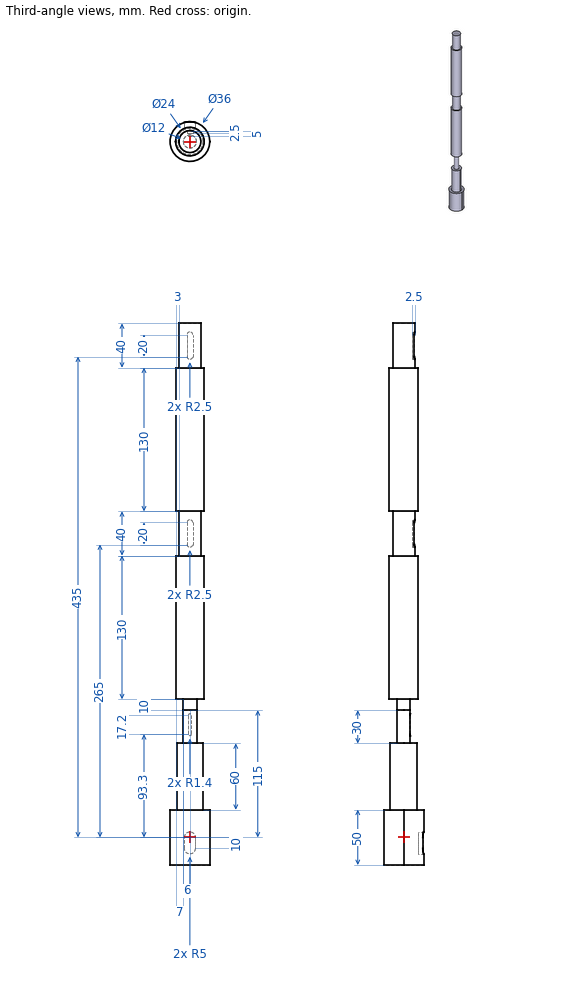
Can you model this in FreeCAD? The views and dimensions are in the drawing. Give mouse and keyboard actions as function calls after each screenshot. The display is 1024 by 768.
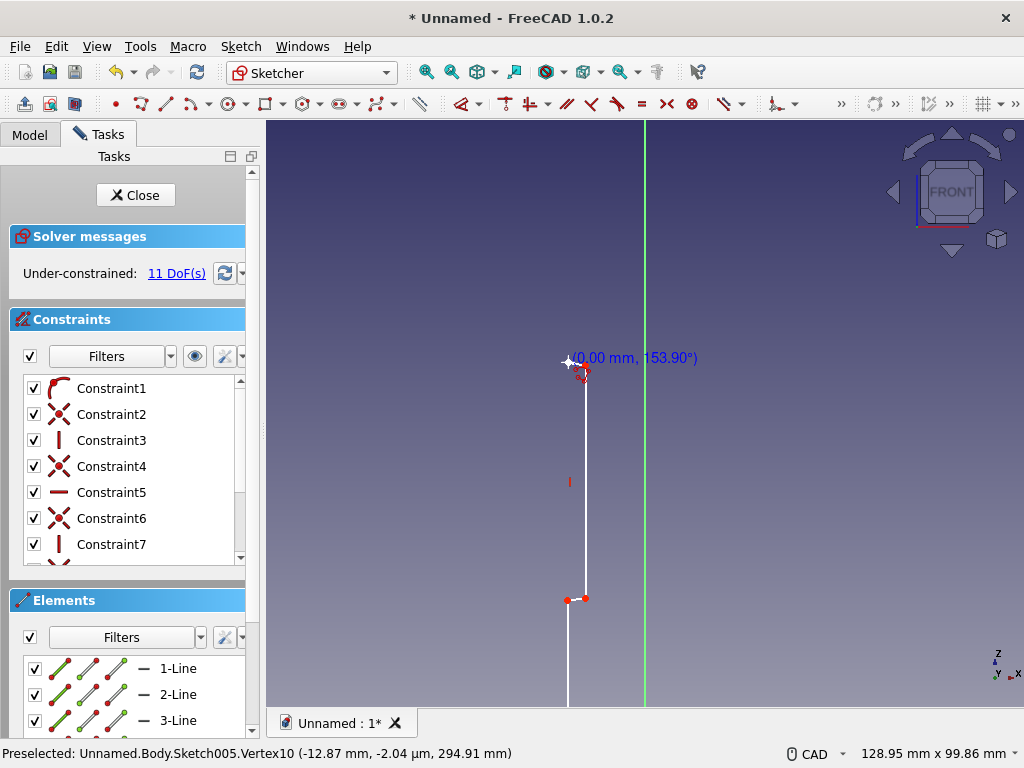
scroll(572, 364, down, 10)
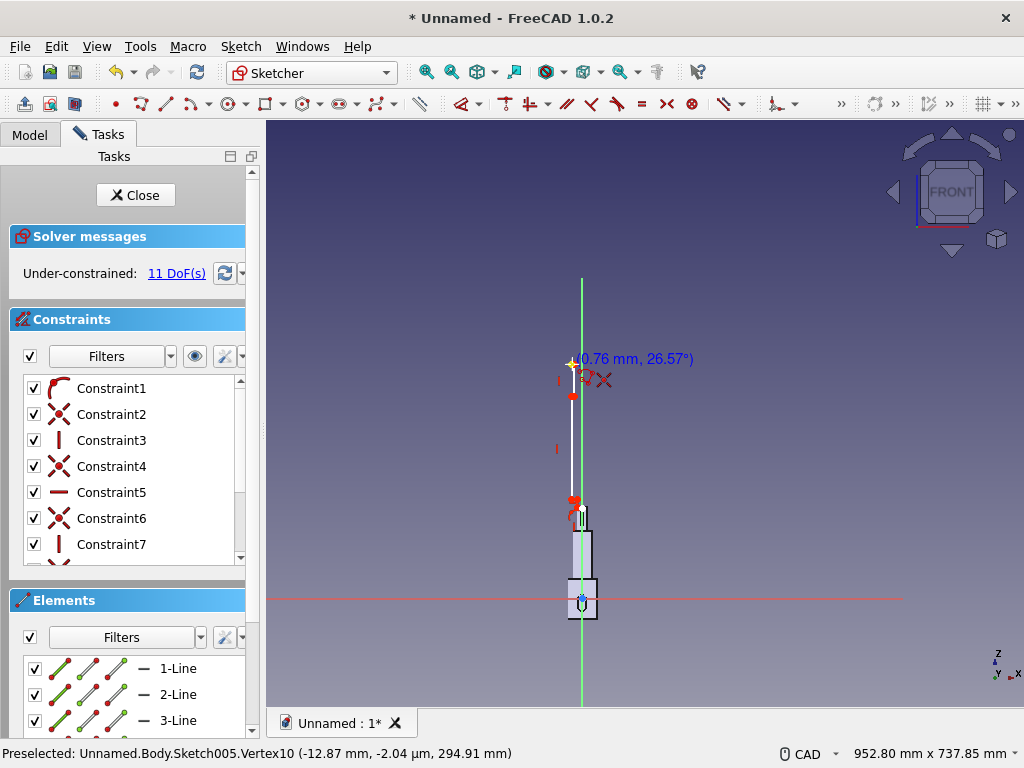
scroll(572, 261, up, 3)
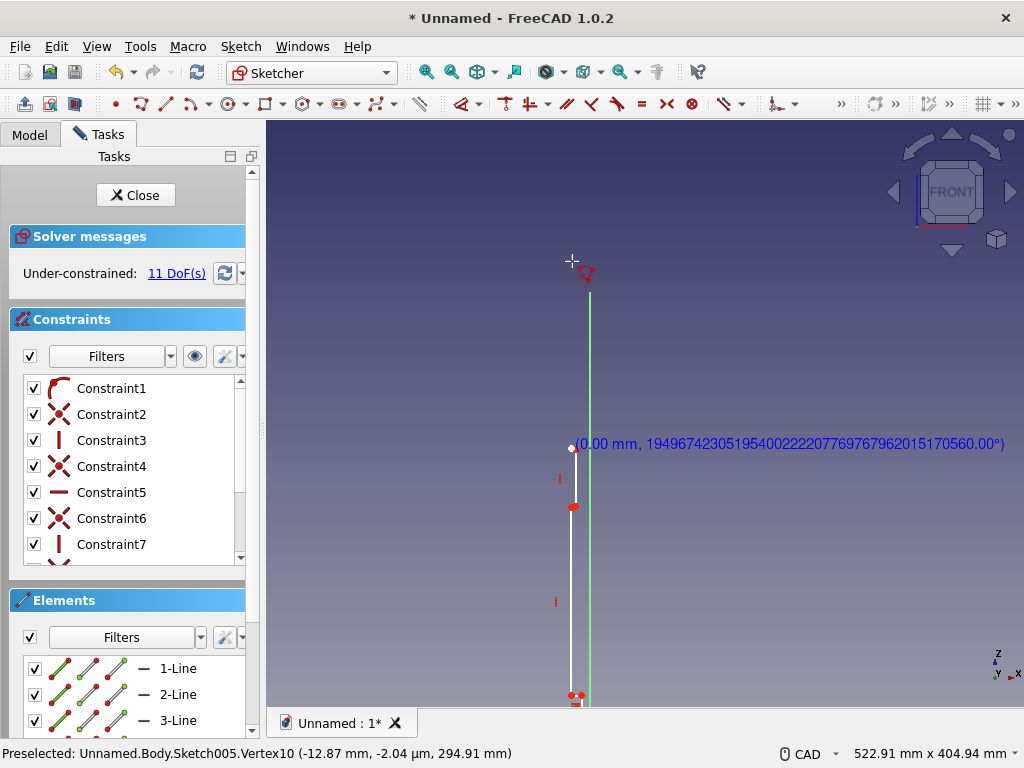
click(571, 261)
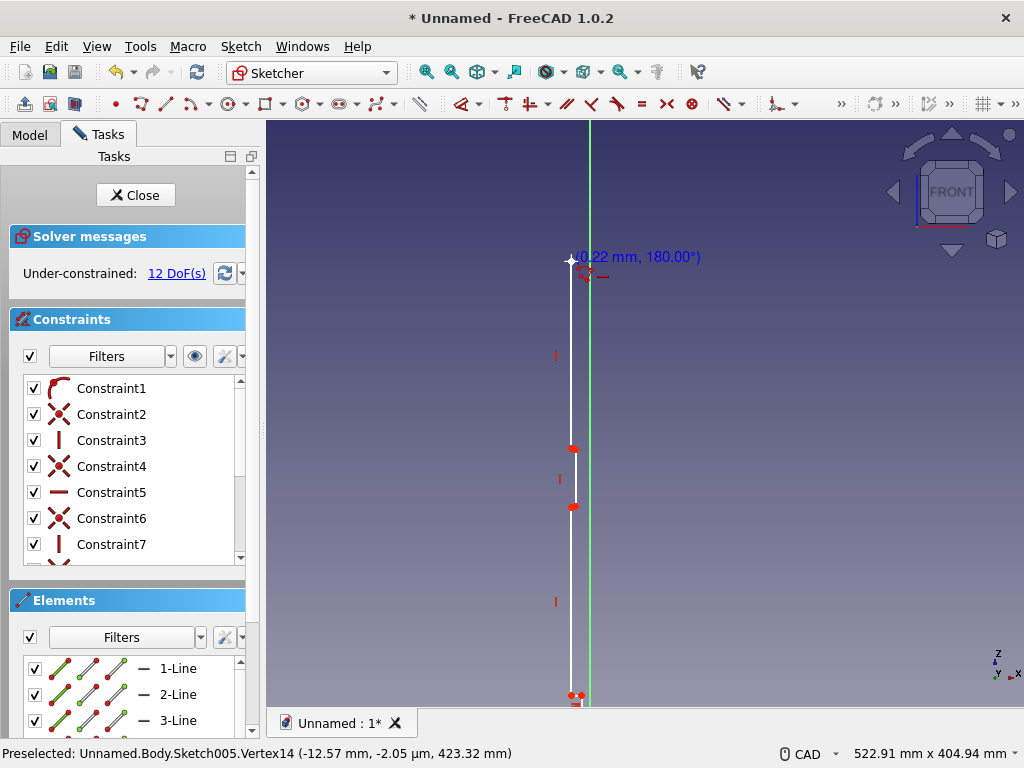
scroll(576, 261, up, 7)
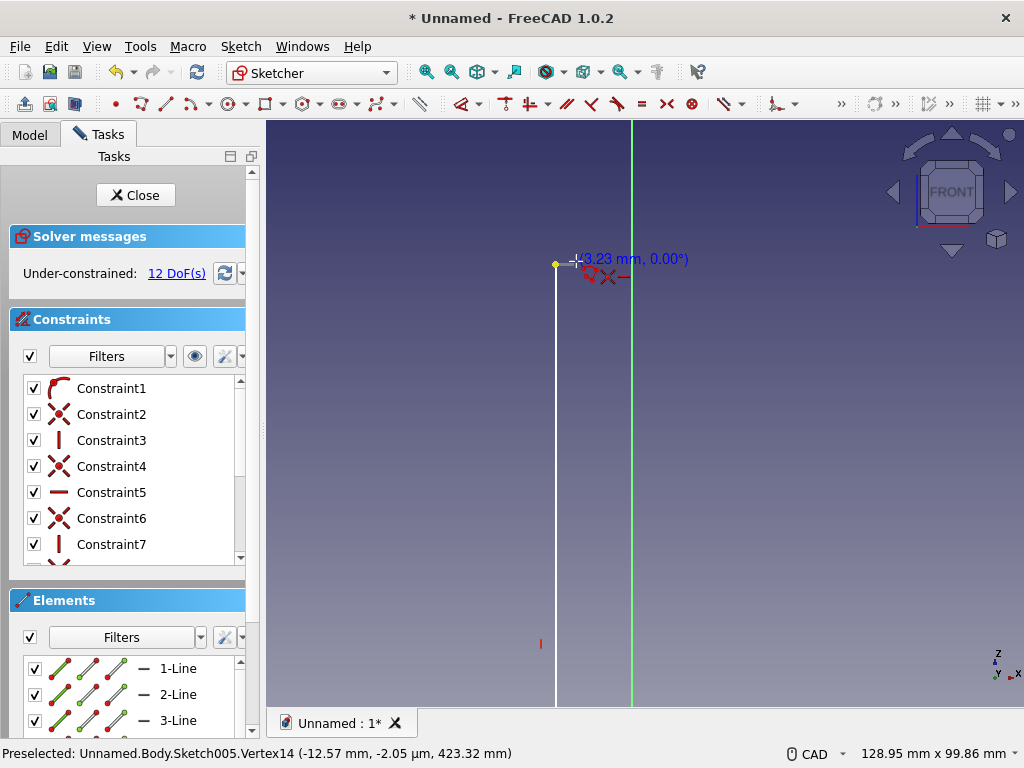
click(574, 260)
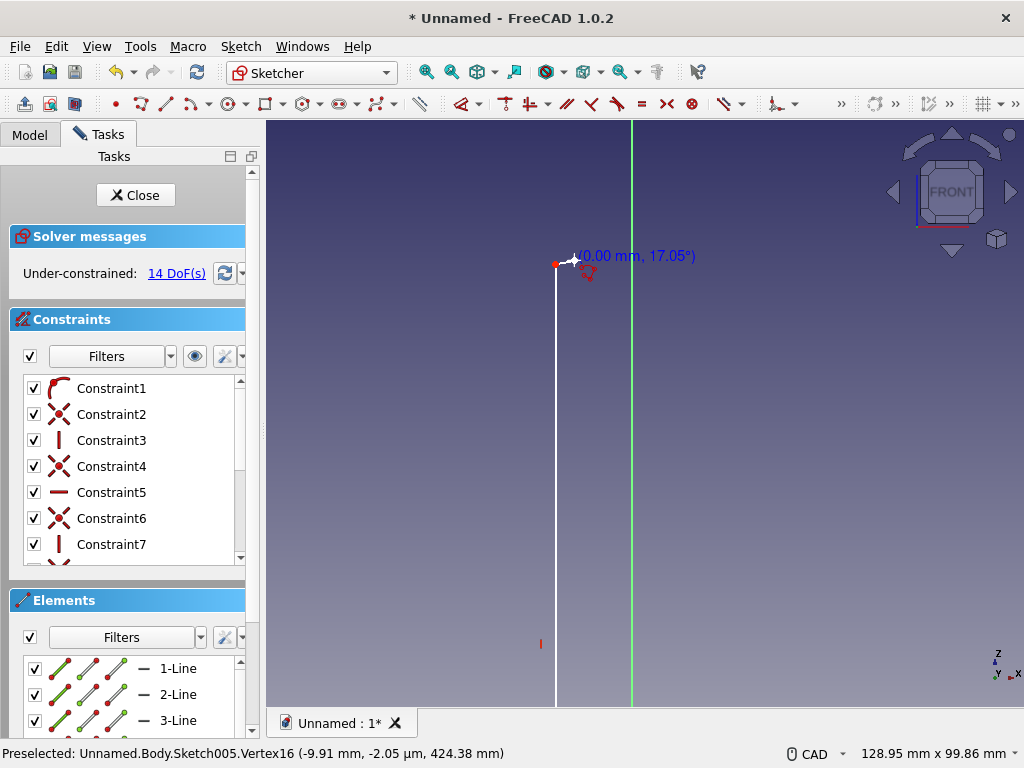
scroll(574, 261, down, 10)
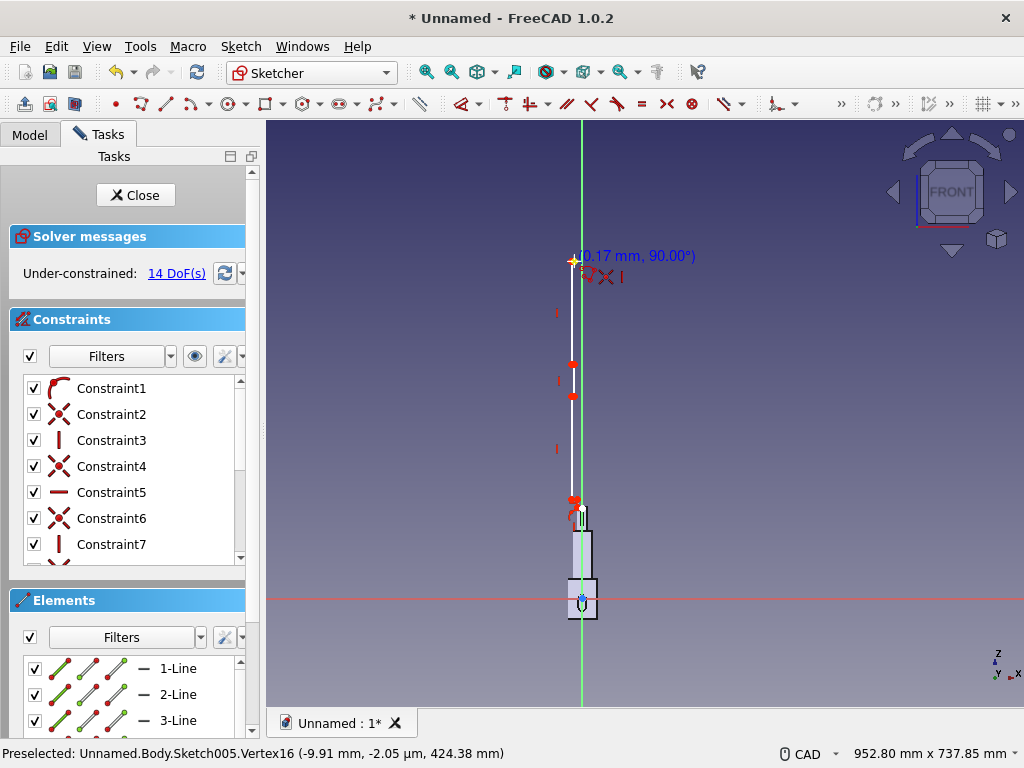
scroll(574, 229, up, 4)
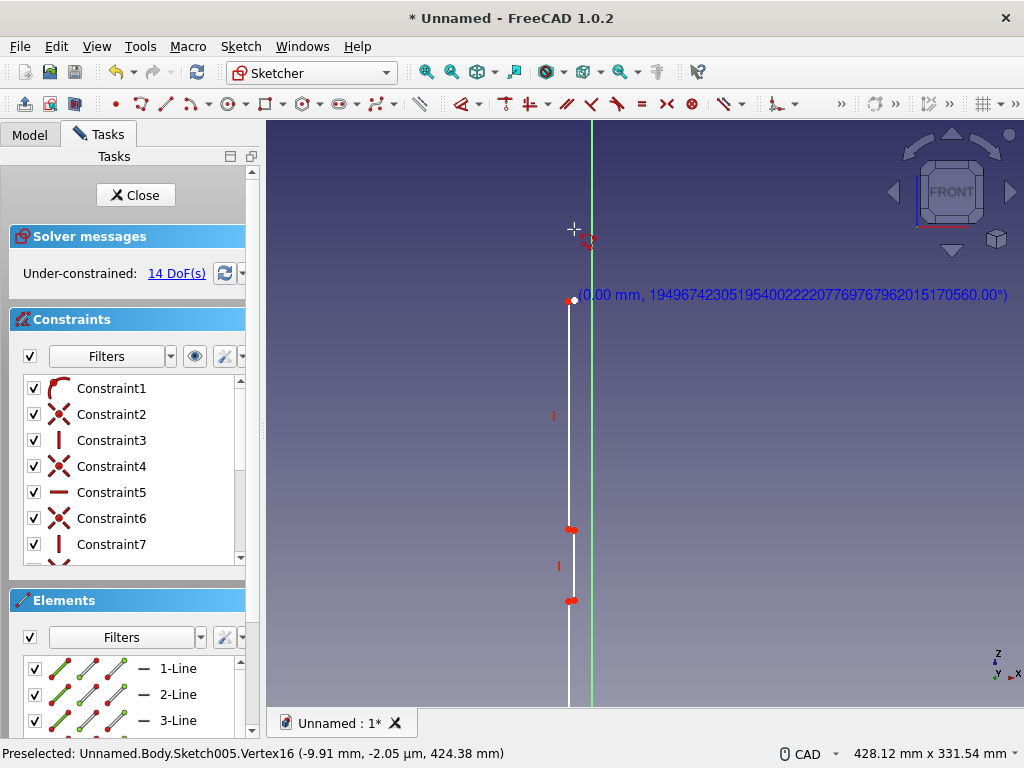
click(574, 229)
click(583, 229)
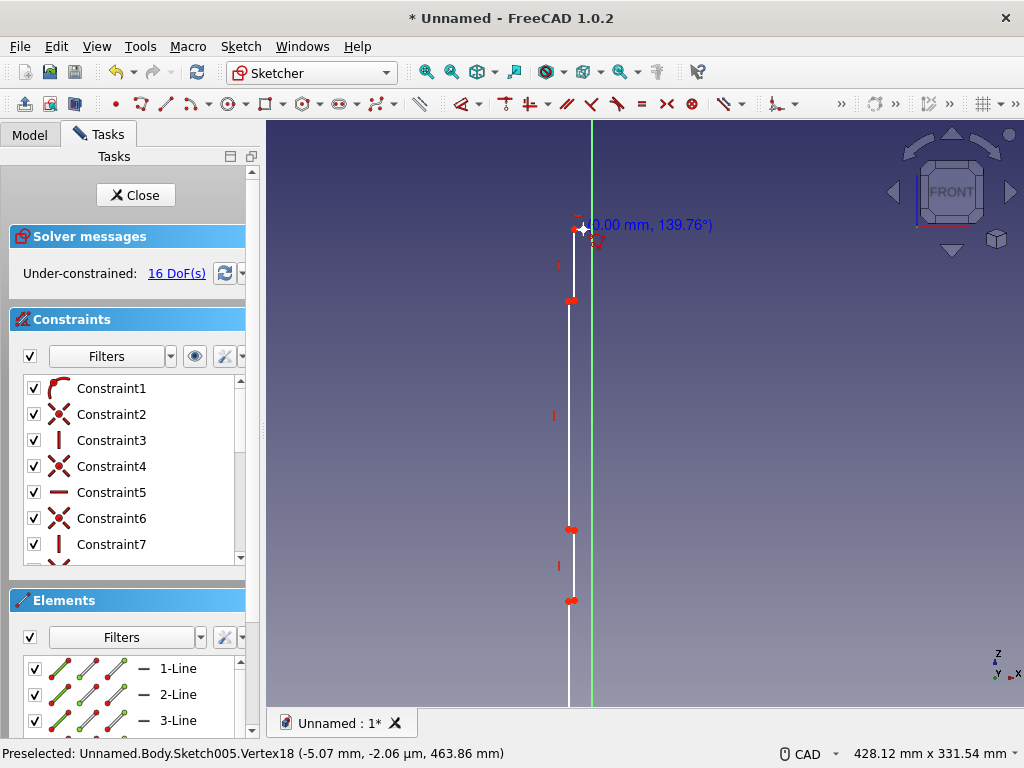
scroll(573, 228, down, 4)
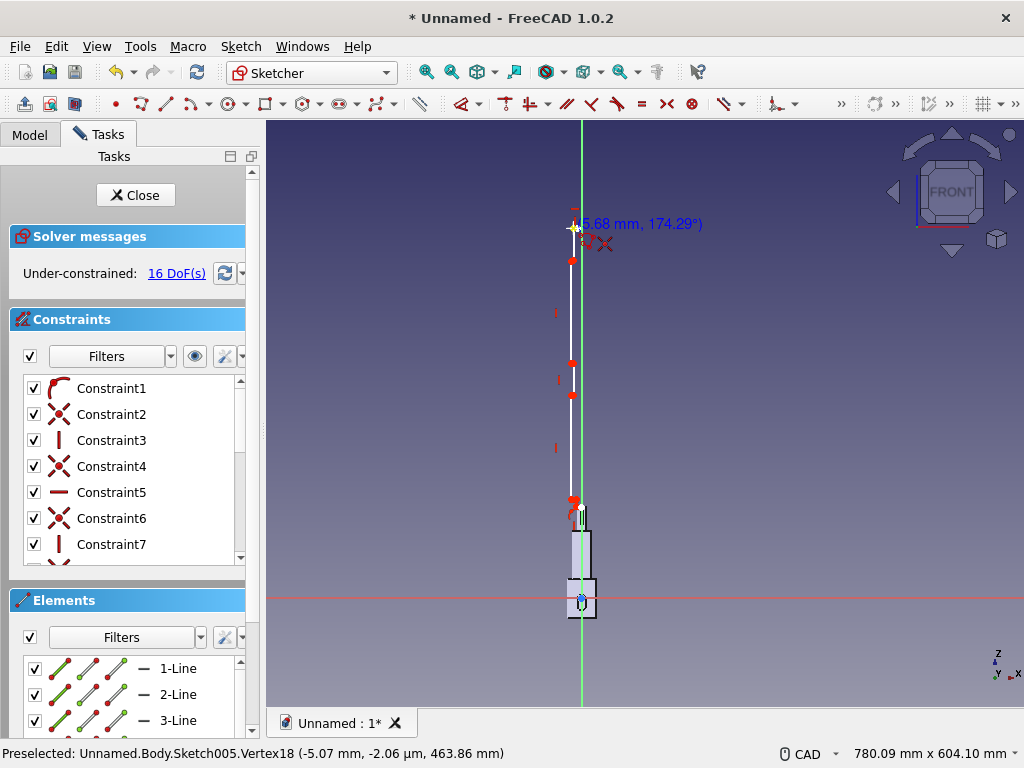
scroll(582, 507, up, 10)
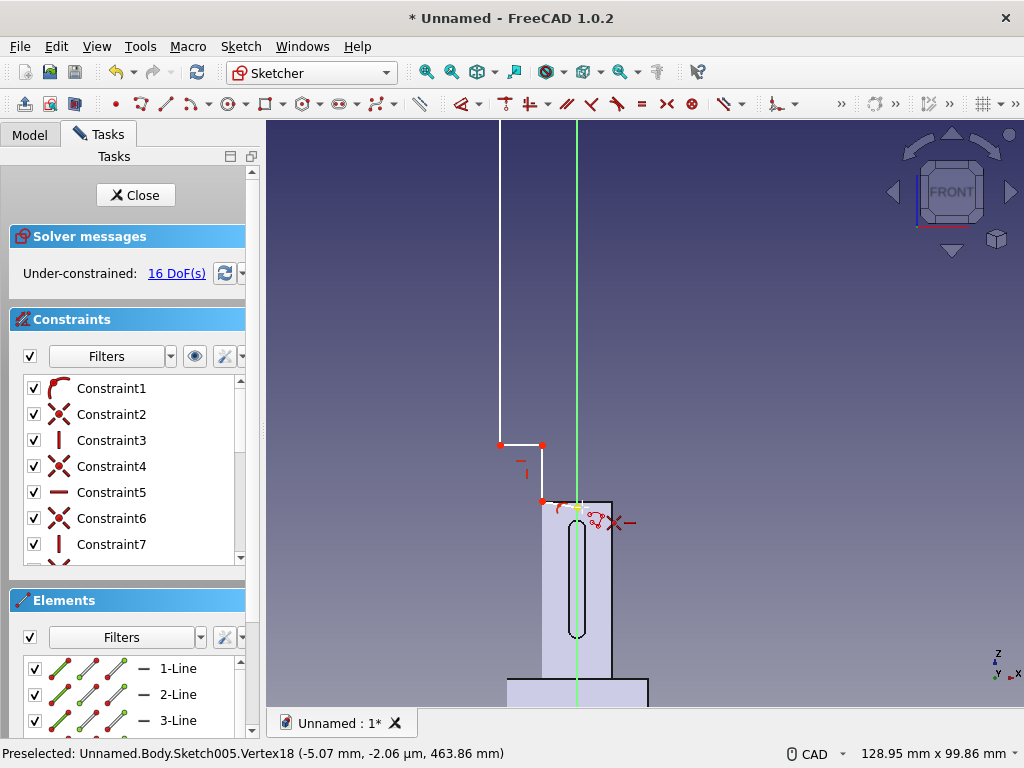
click(577, 507)
key(Escape)
key(Escape)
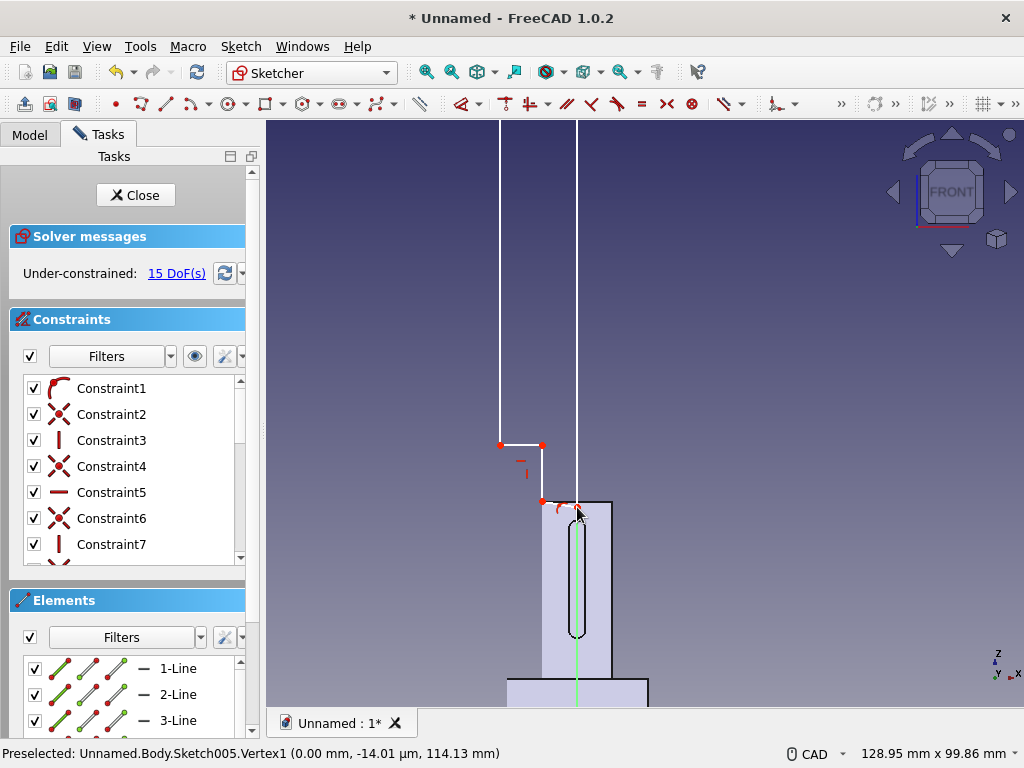
scroll(567, 506, up, 2)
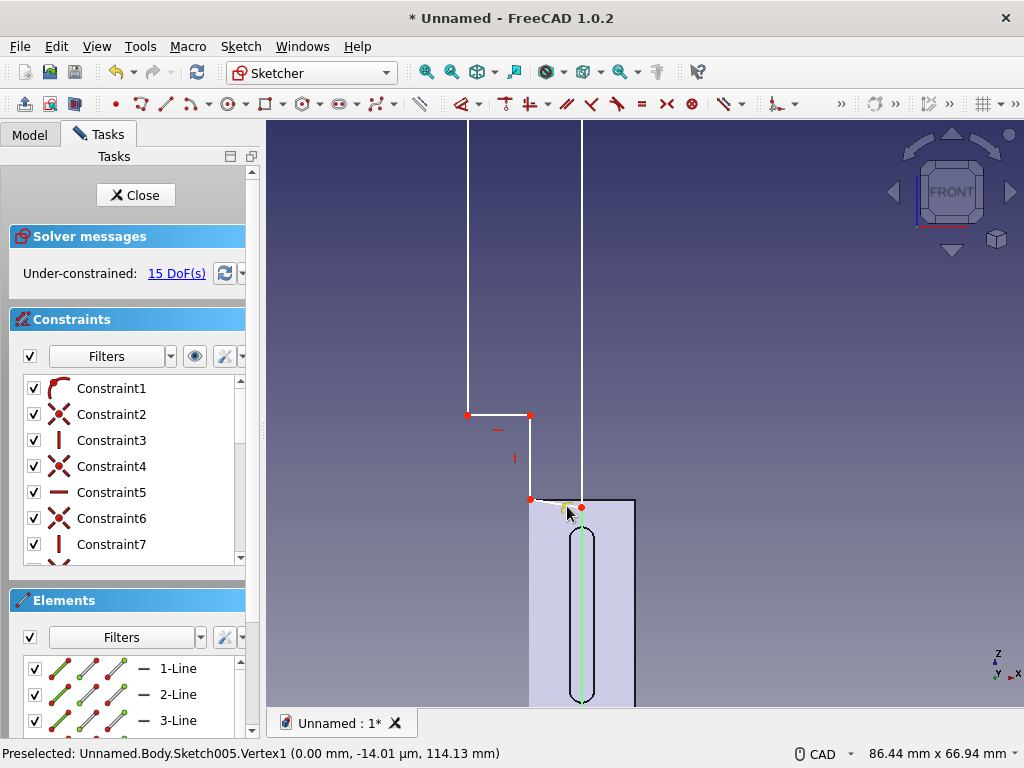
click(546, 502)